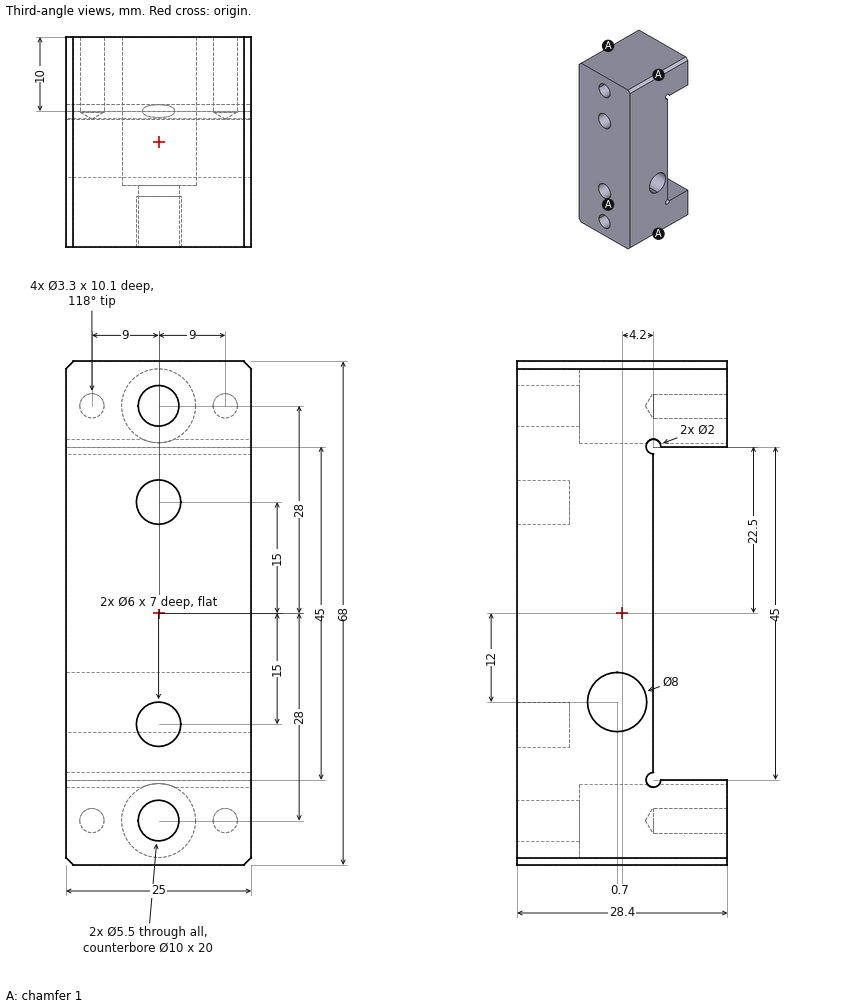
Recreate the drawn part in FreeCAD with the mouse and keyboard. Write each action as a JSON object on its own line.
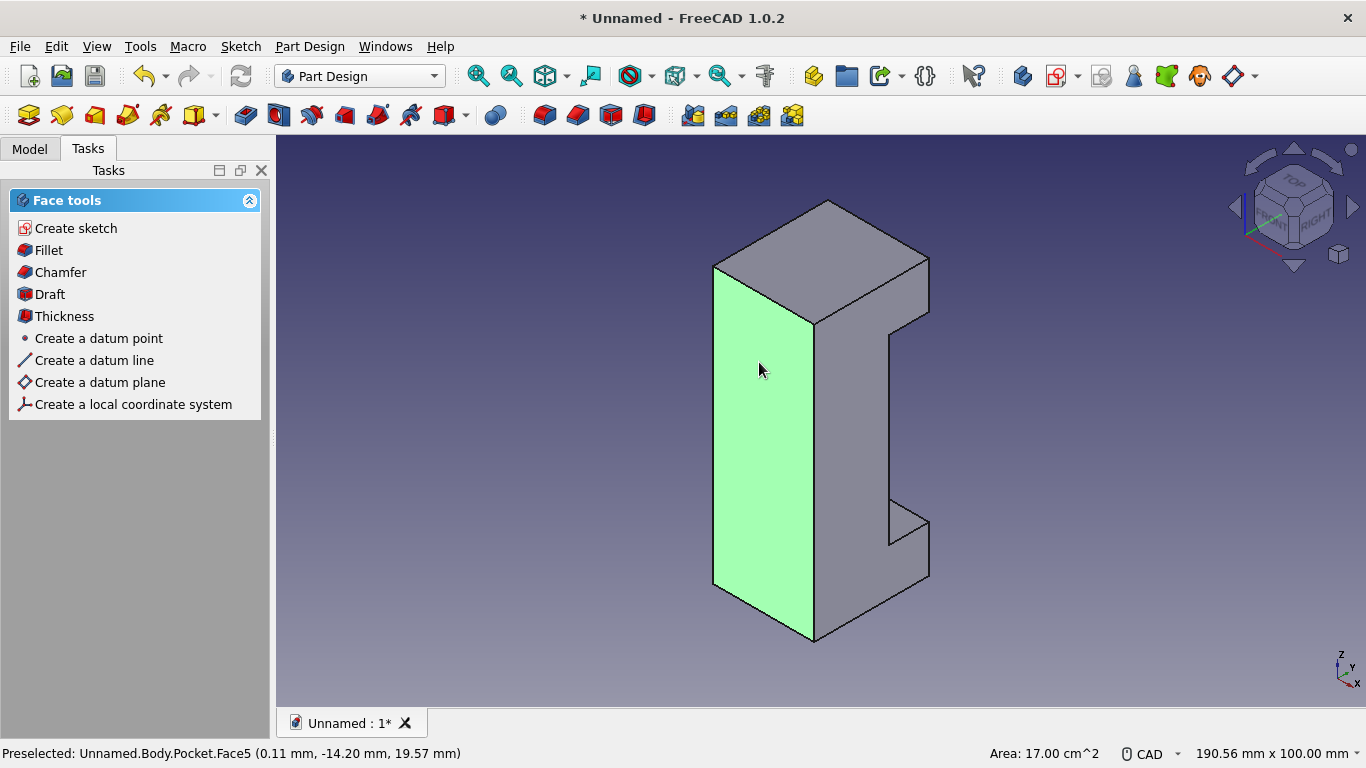
{"action": "left_click", "coordinate": [1056, 76]}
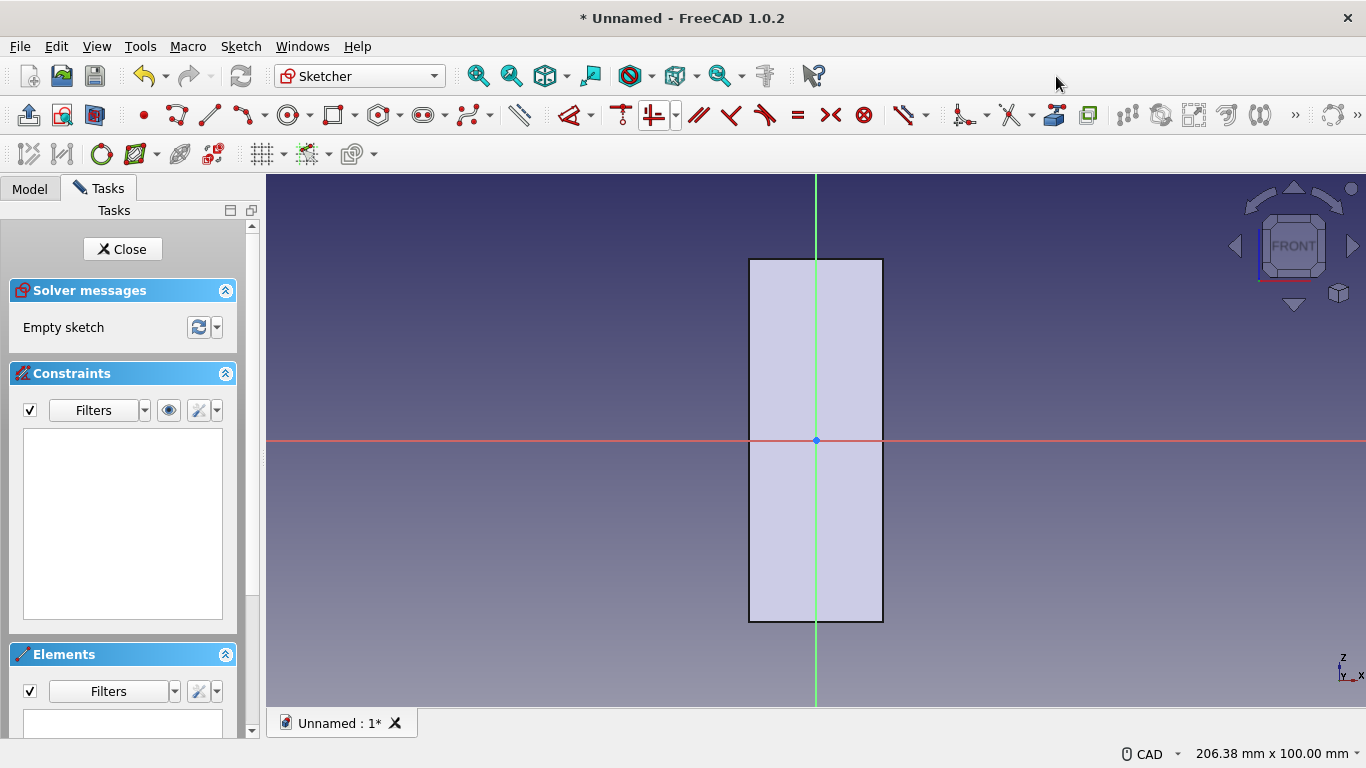
{"action": "scroll", "coordinate": [899, 441], "scroll_direction": "up", "scroll_amount": 3}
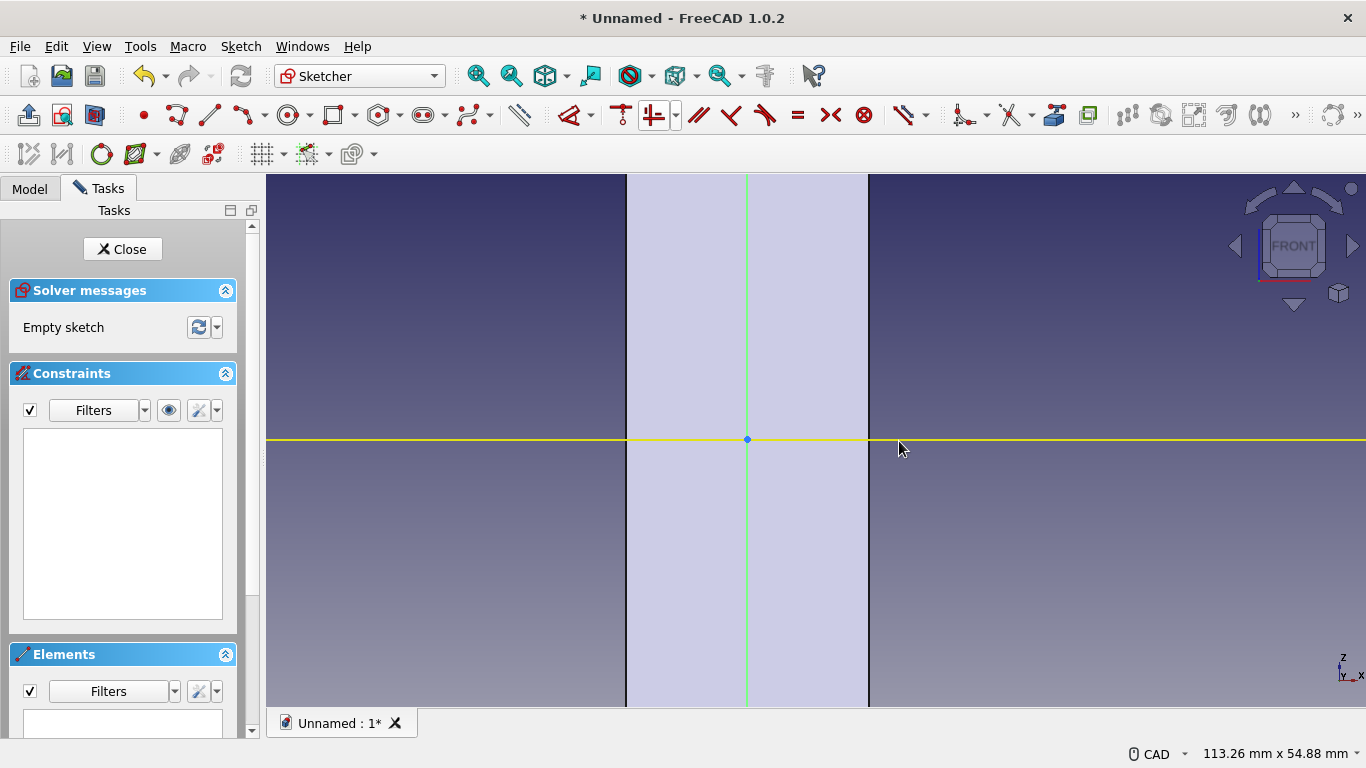
{"action": "key", "text": "g c"}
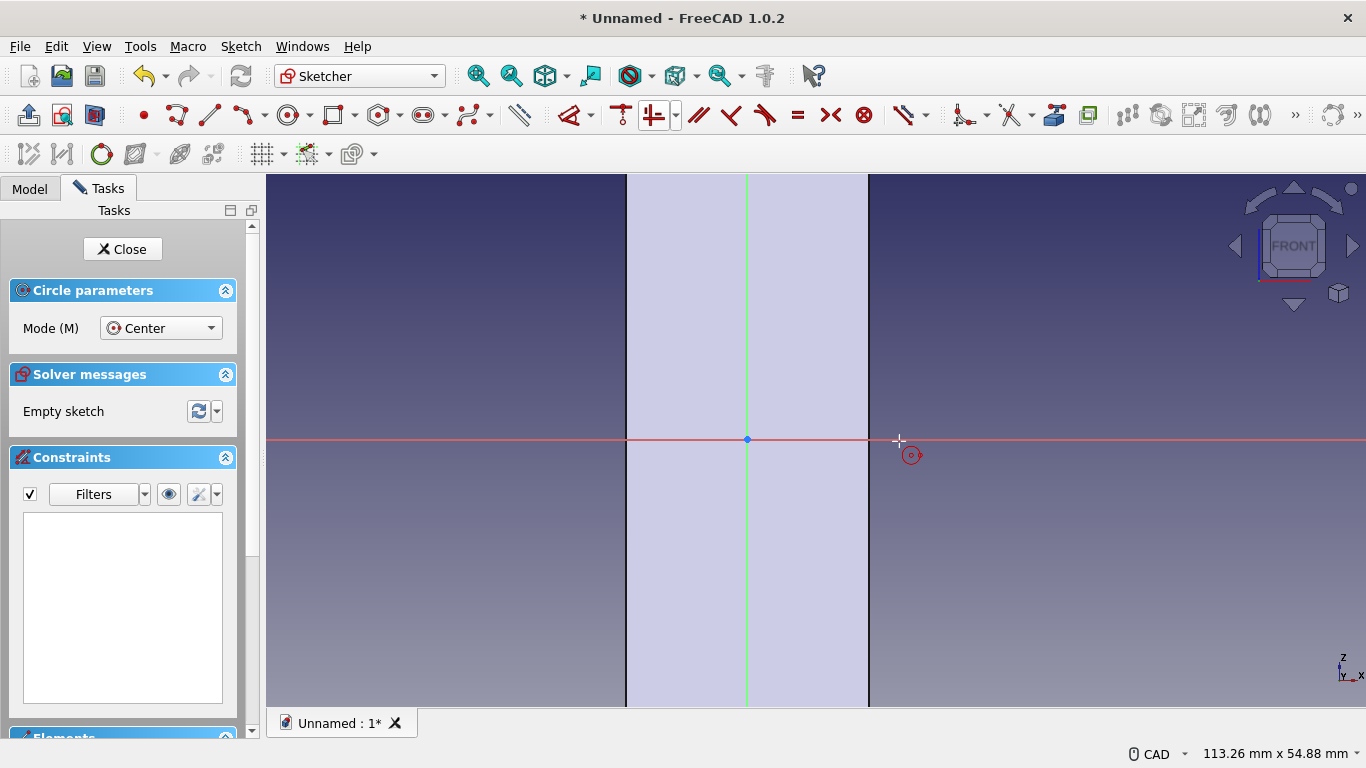
{"action": "left_click", "coordinate": [747, 585]}
{"action": "left_click", "coordinate": [768, 565]}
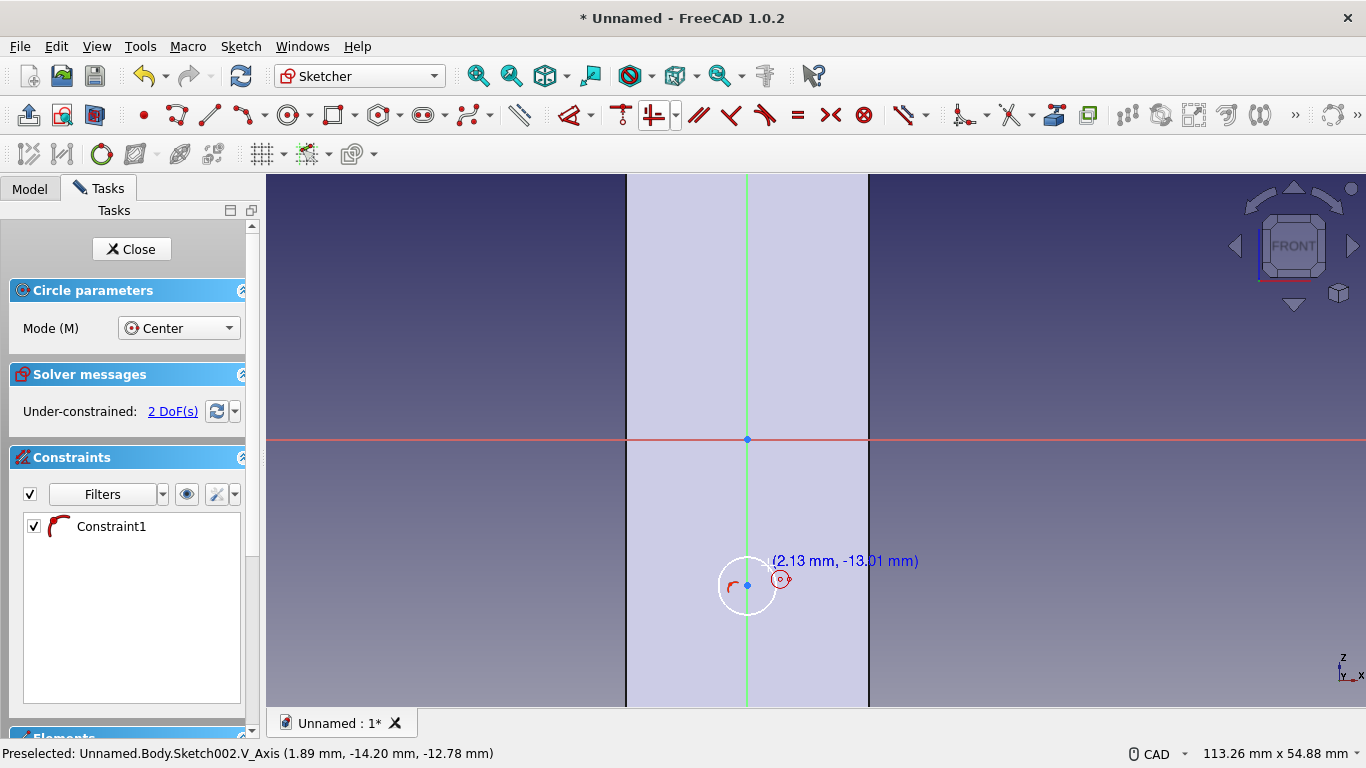
{"action": "left_click", "coordinate": [747, 294]}
{"action": "left_click", "coordinate": [768, 273]}
{"action": "key", "text": "Escape"}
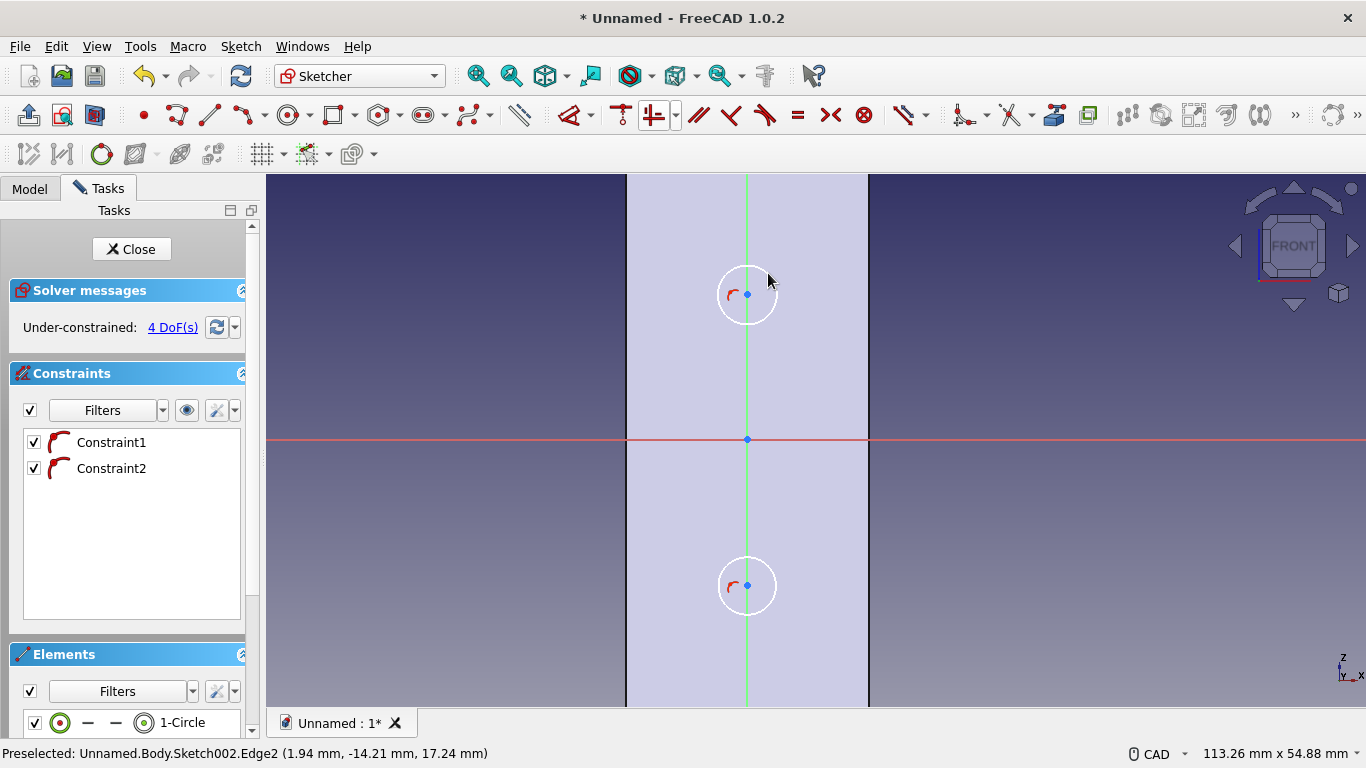
{"action": "left_click", "coordinate": [768, 566]}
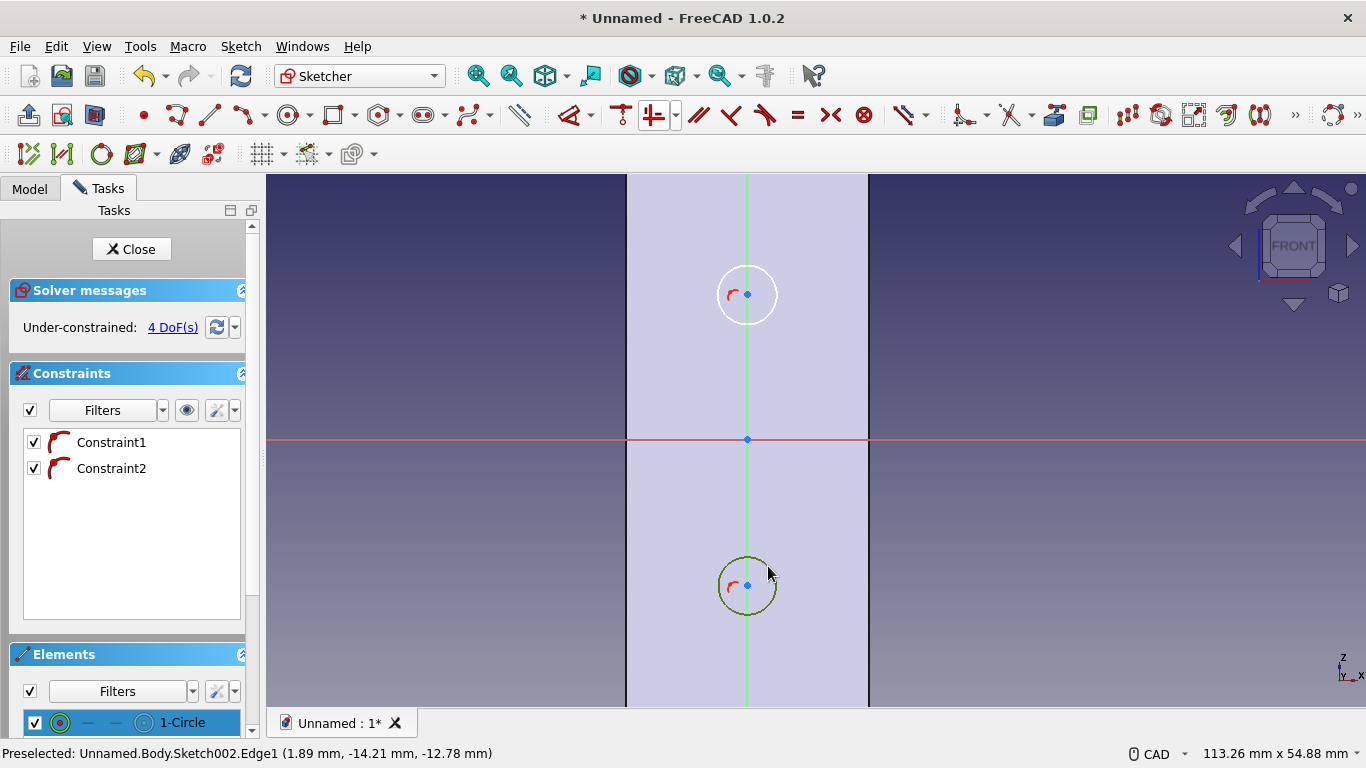
{"action": "left_click", "coordinate": [768, 274]}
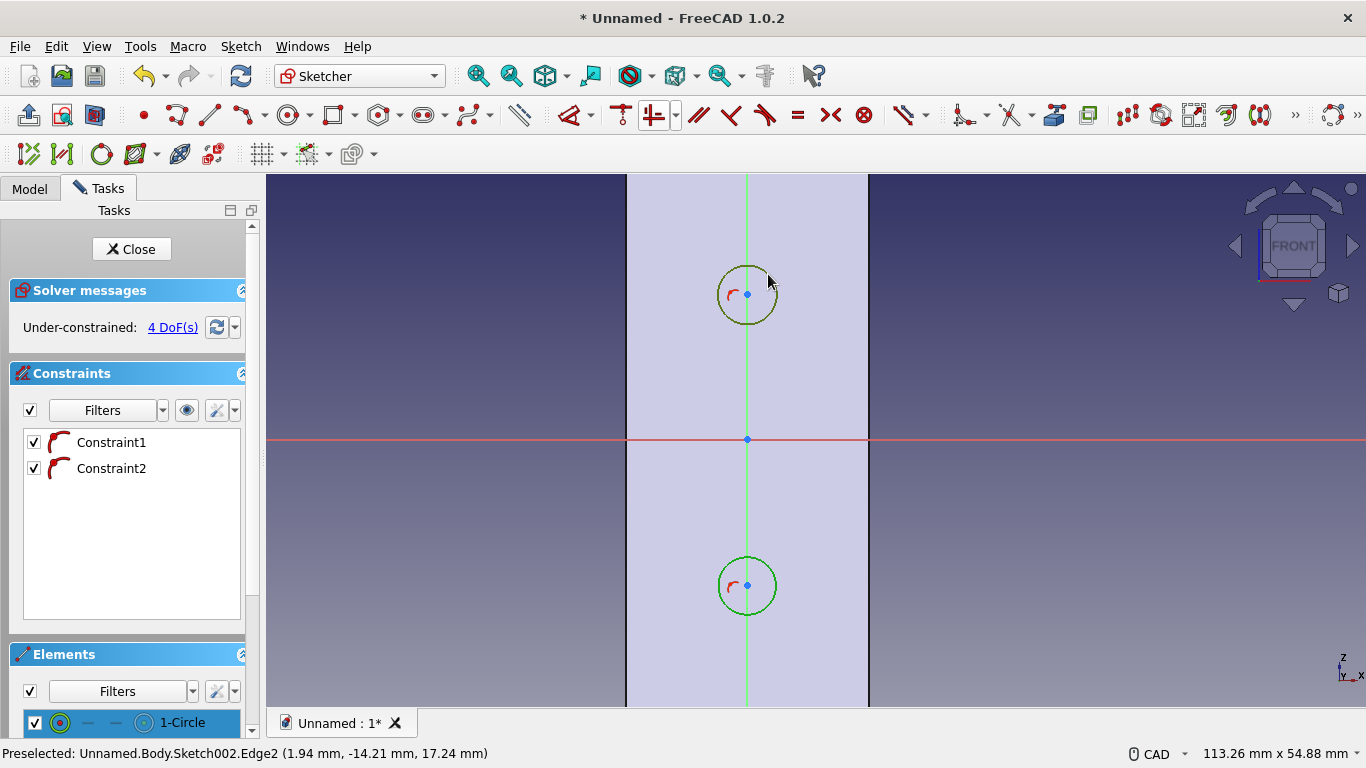
{"action": "key", "text": "e"}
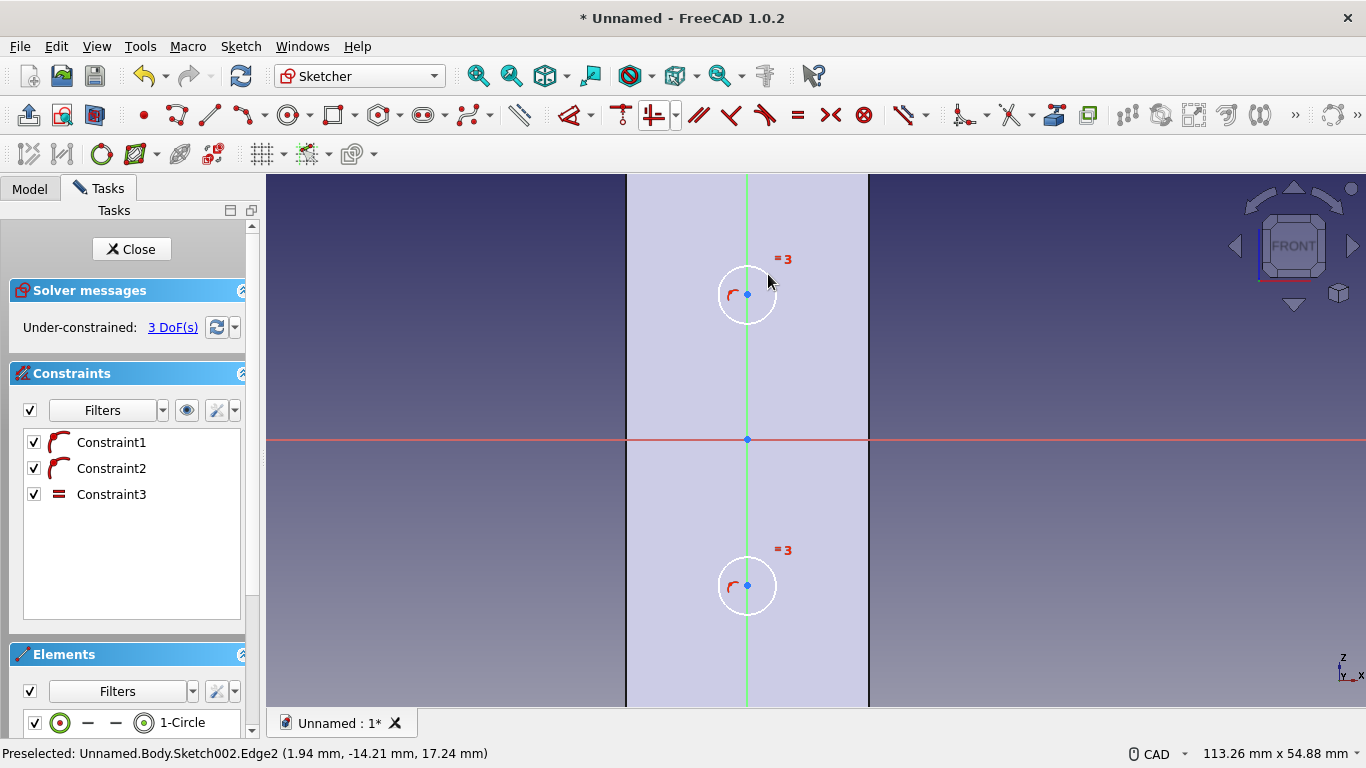
{"action": "key", "text": "d"}